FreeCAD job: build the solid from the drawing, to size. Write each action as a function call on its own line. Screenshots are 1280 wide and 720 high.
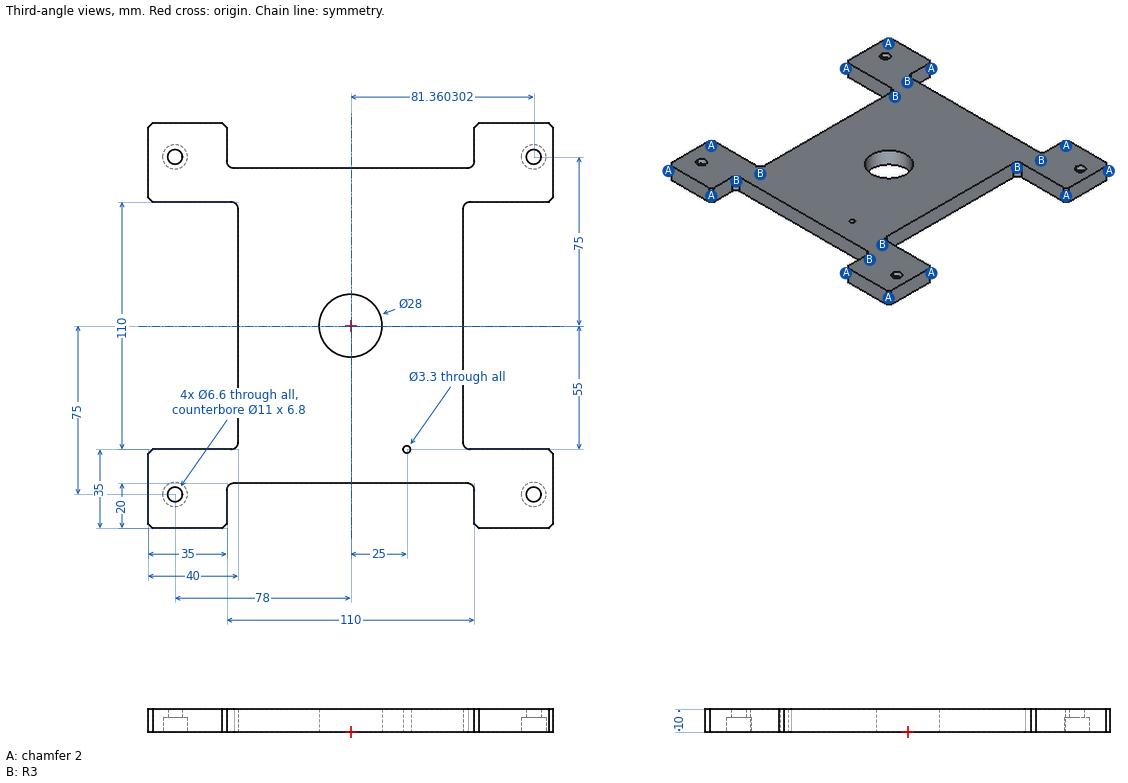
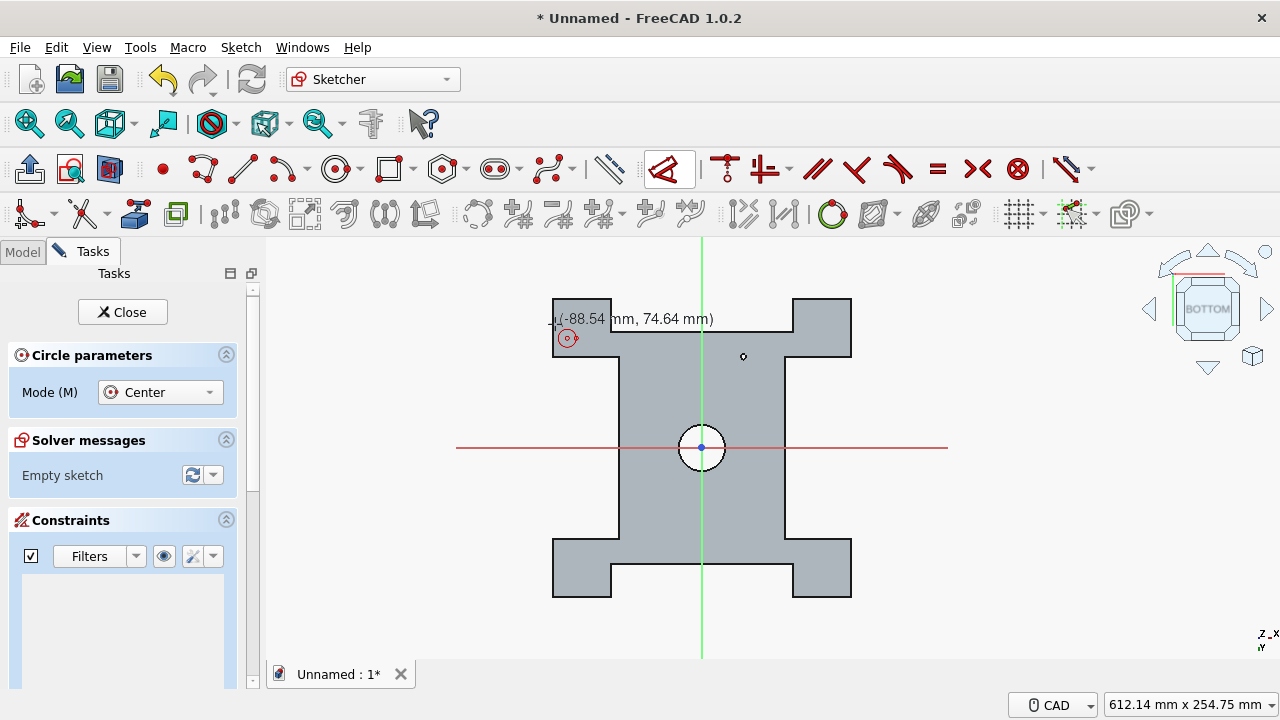
click(573, 324)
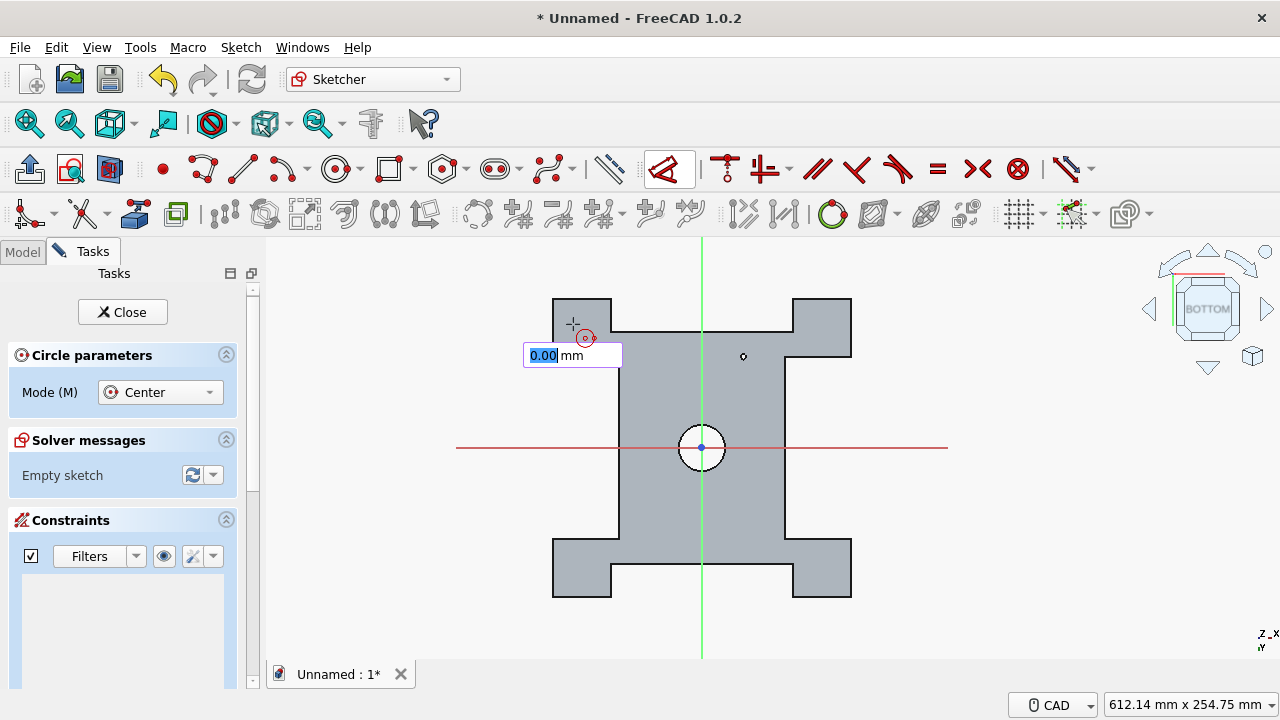
scroll(577, 320, up, 6)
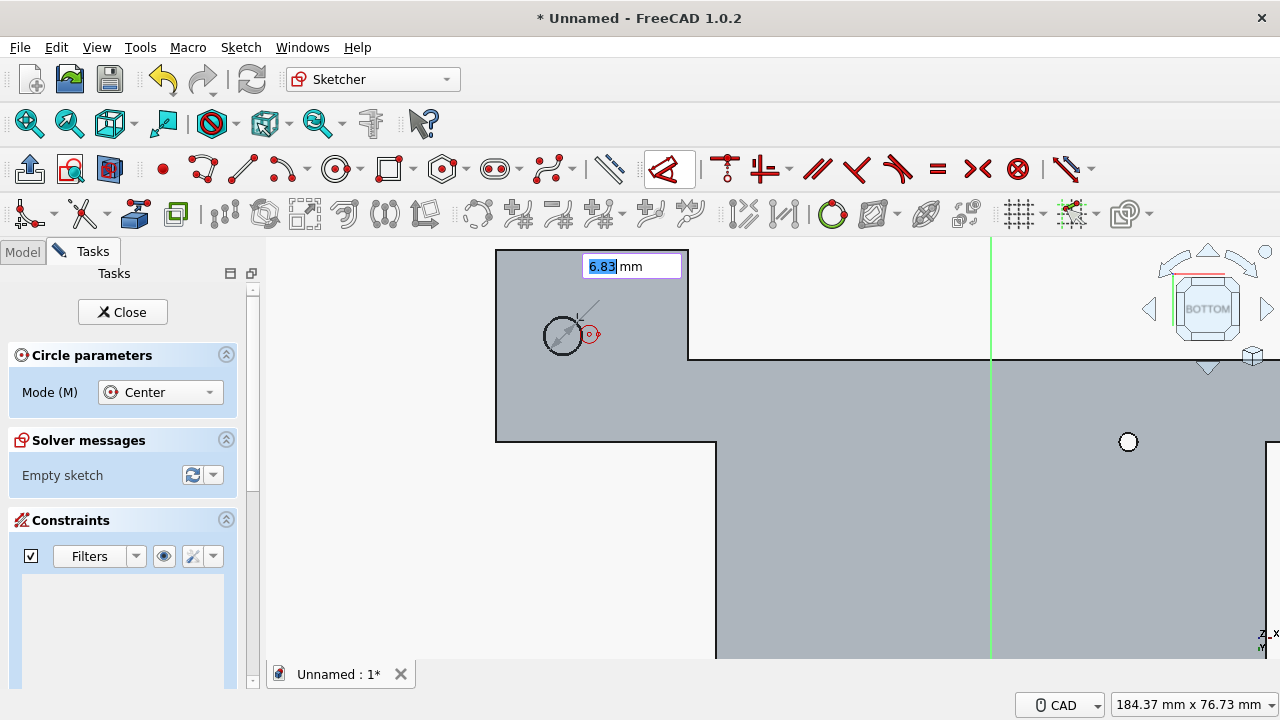
click(575, 319)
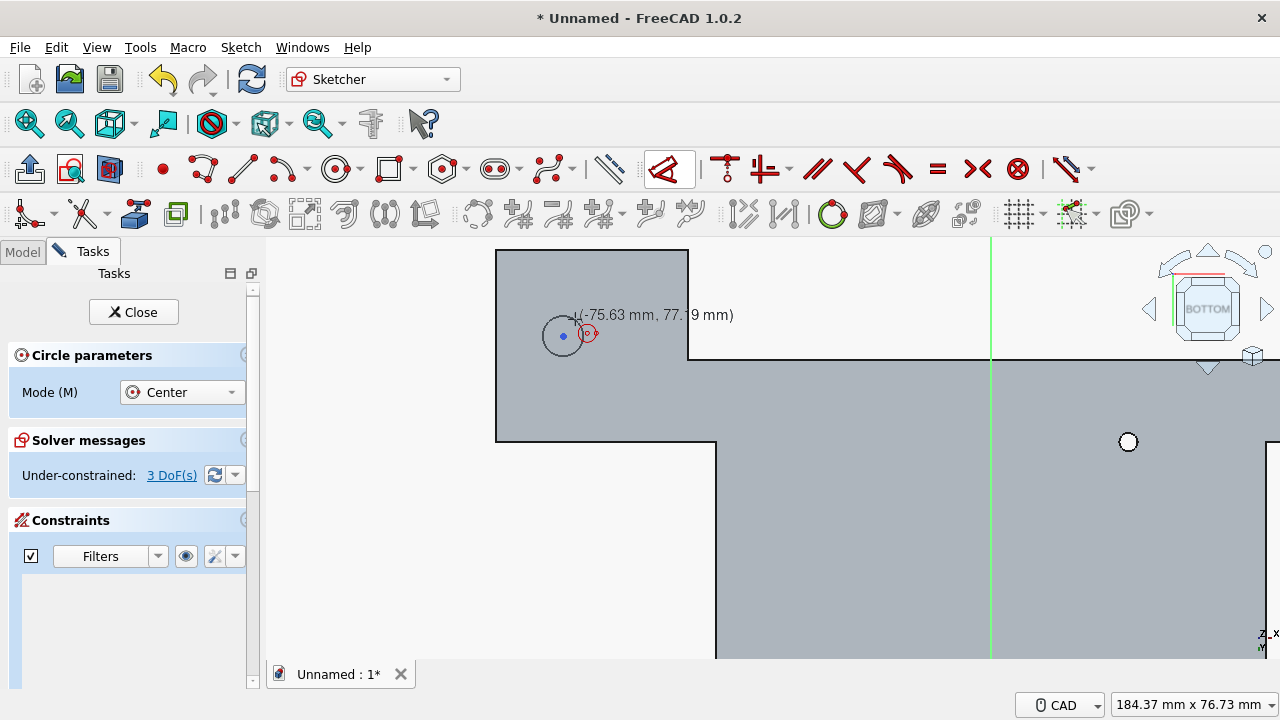
scroll(577, 320, down, 6)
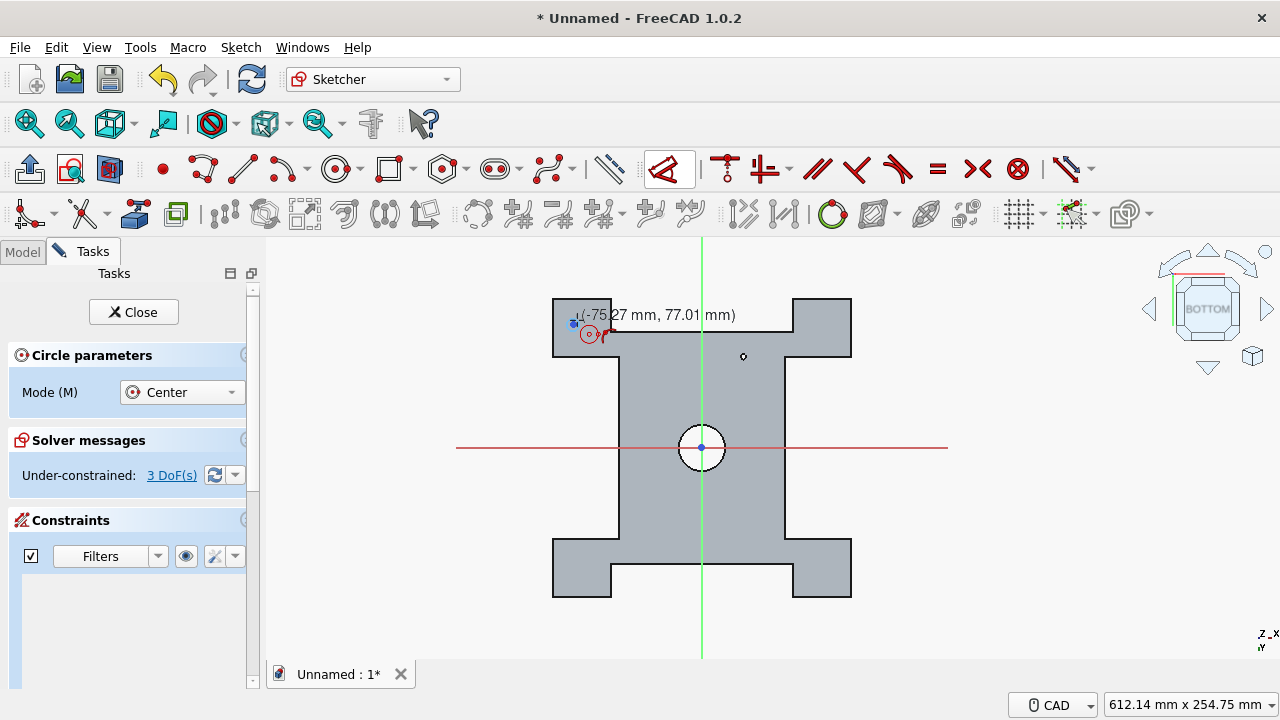
scroll(573, 572, up, 8)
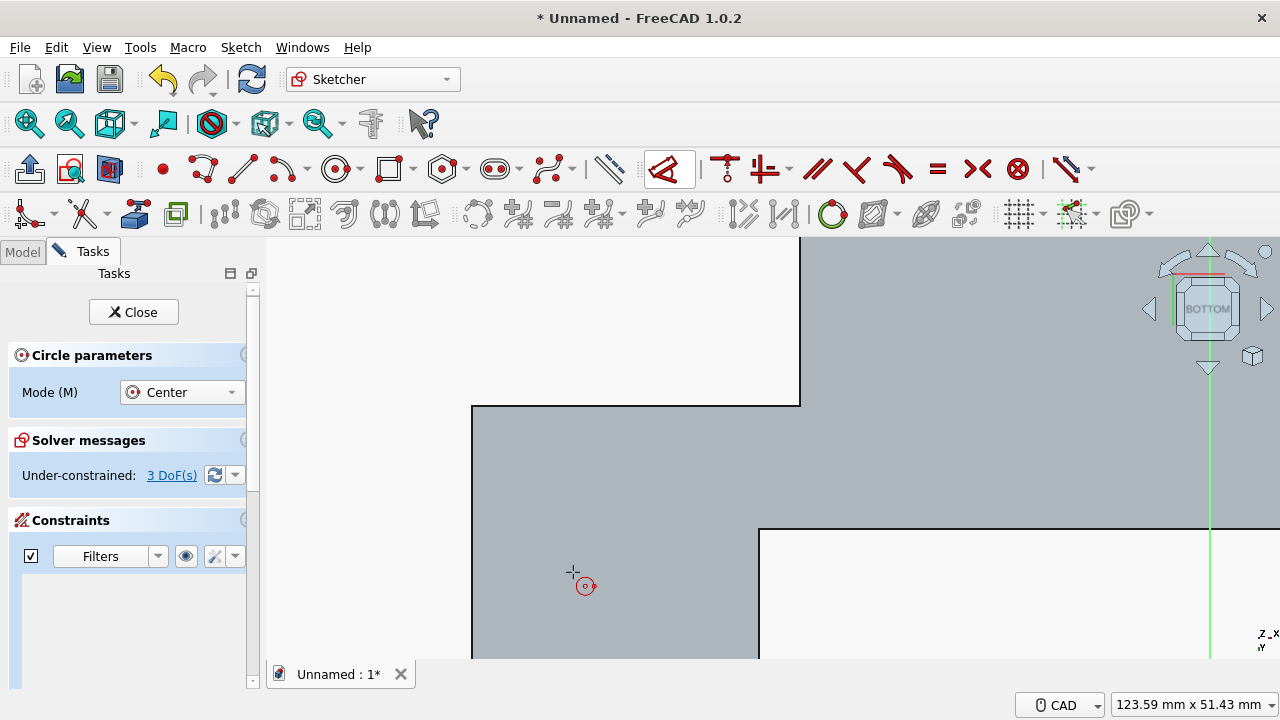
scroll(573, 573, down, 8)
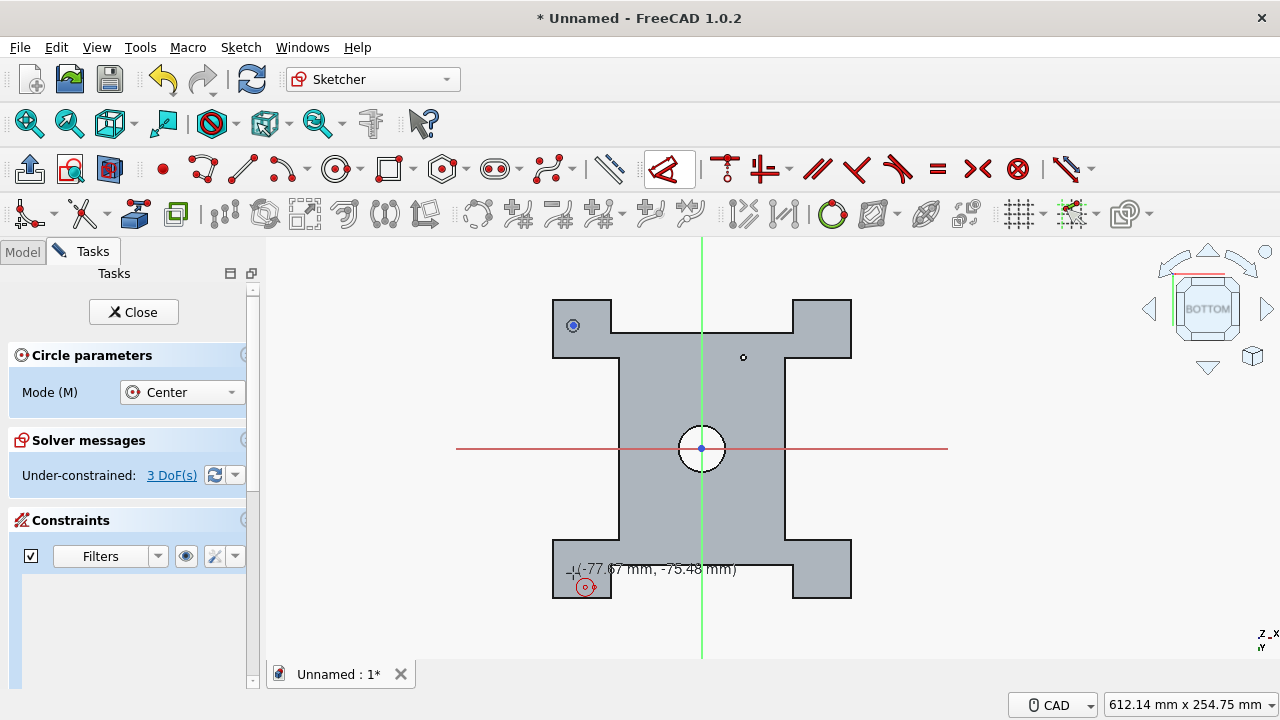
click(573, 573)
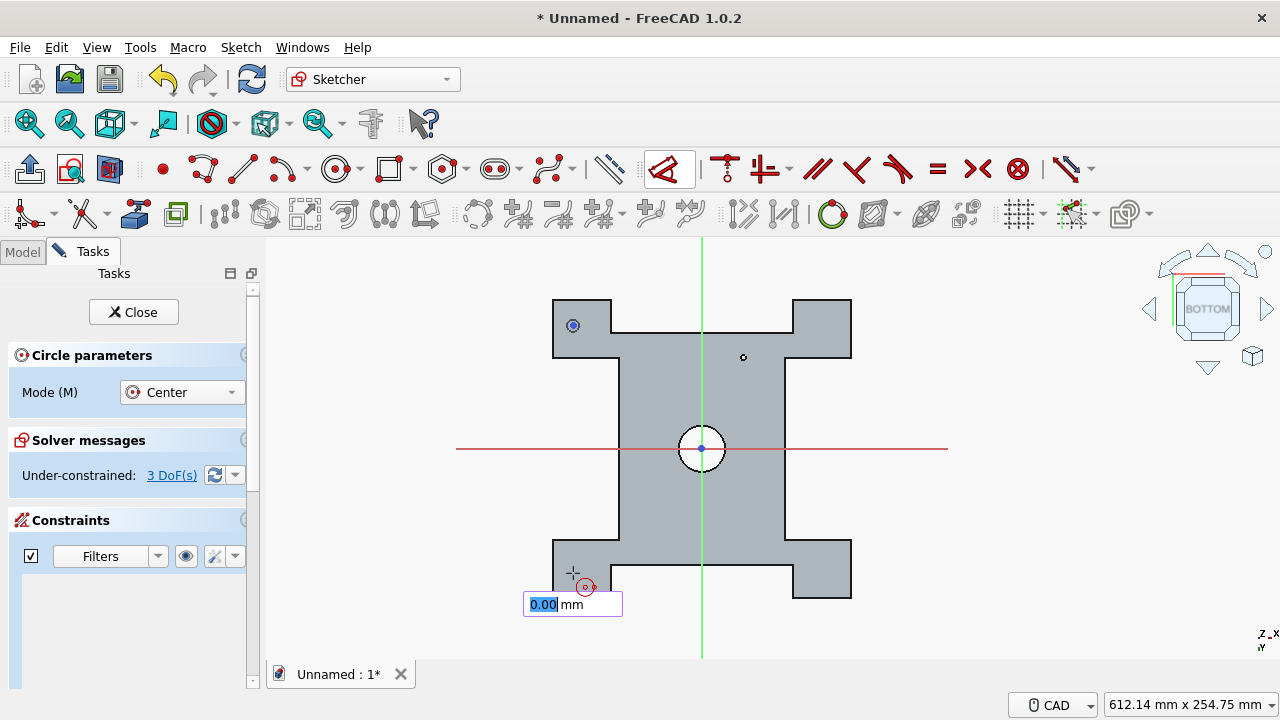
scroll(577, 569, up, 6)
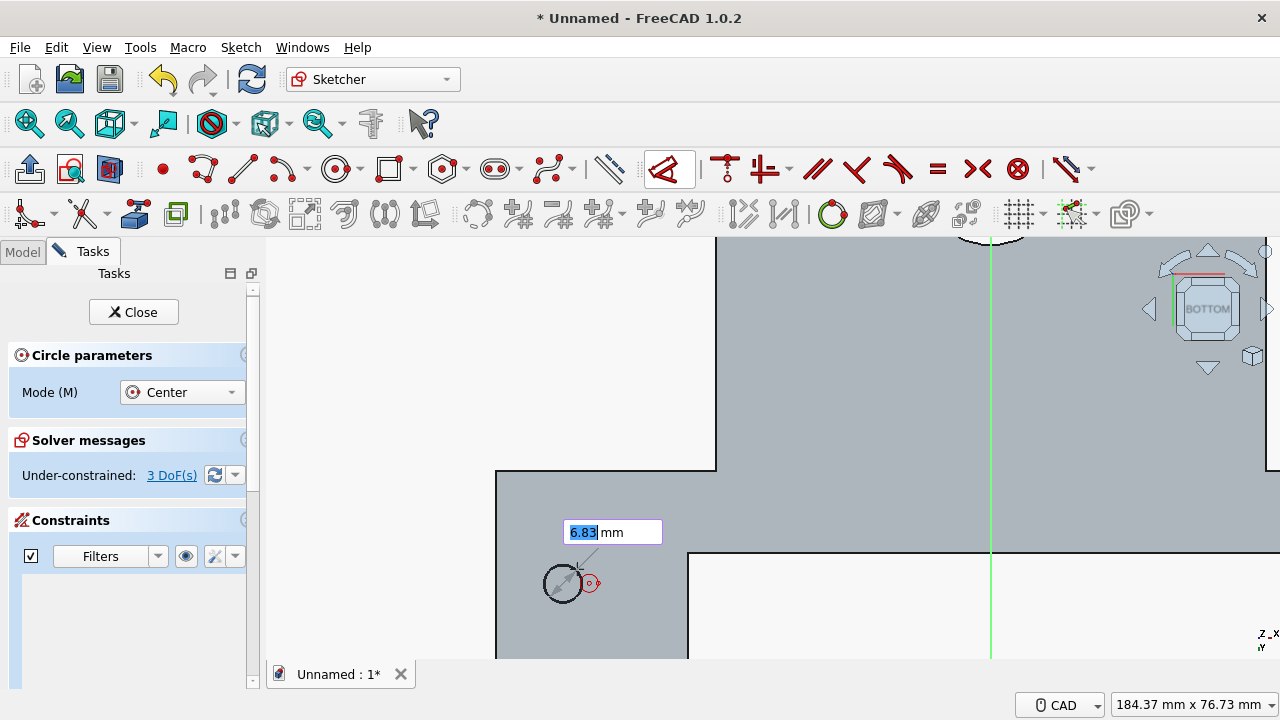
click(575, 568)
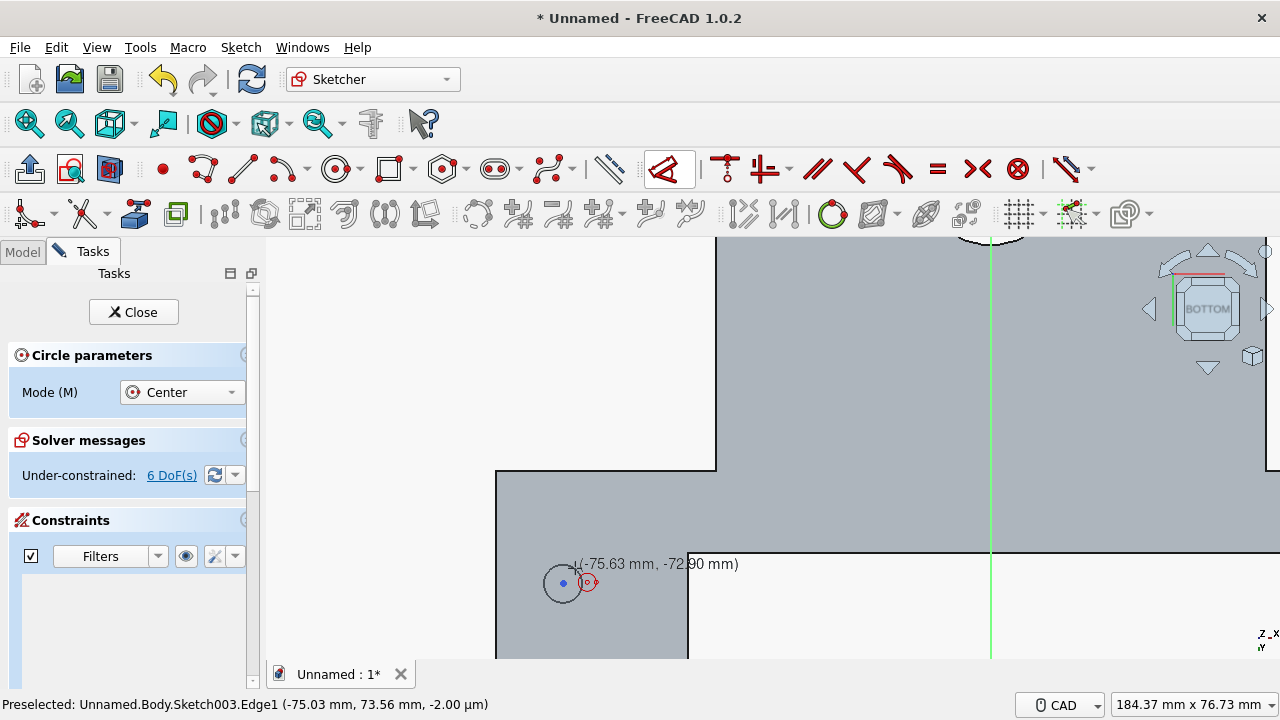
scroll(577, 569, down, 6)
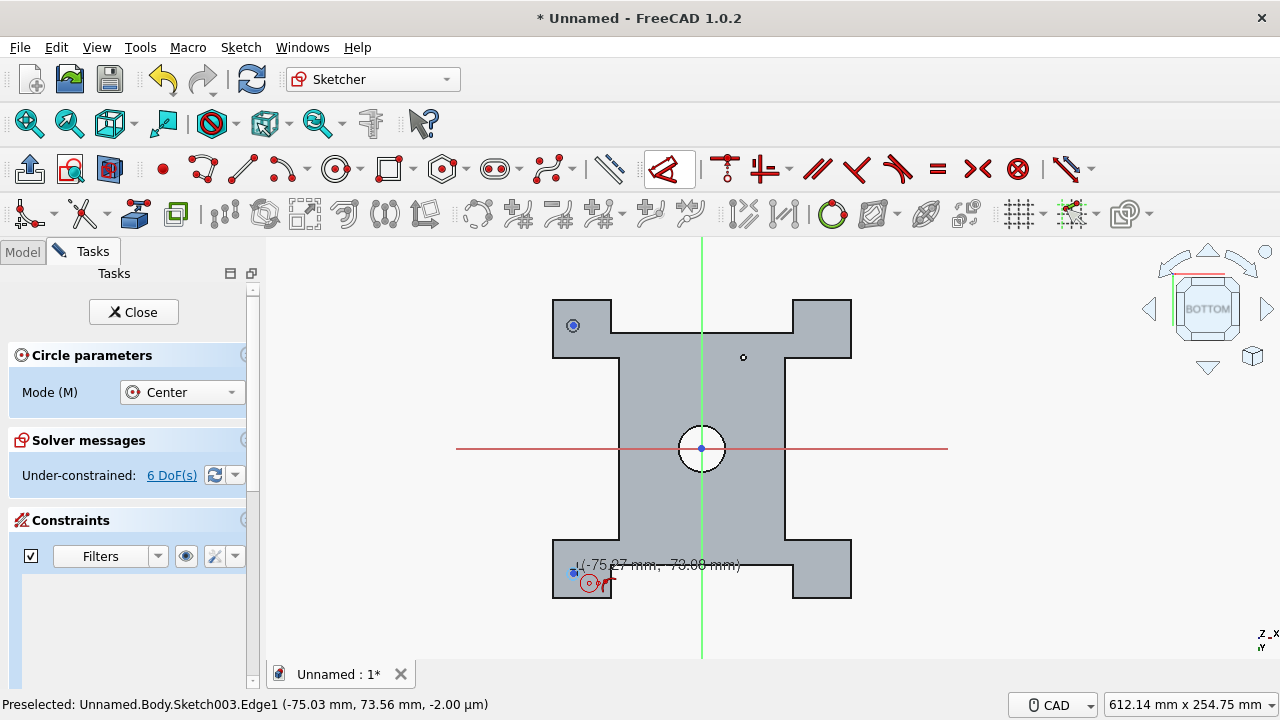
scroll(837, 573, up, 8)